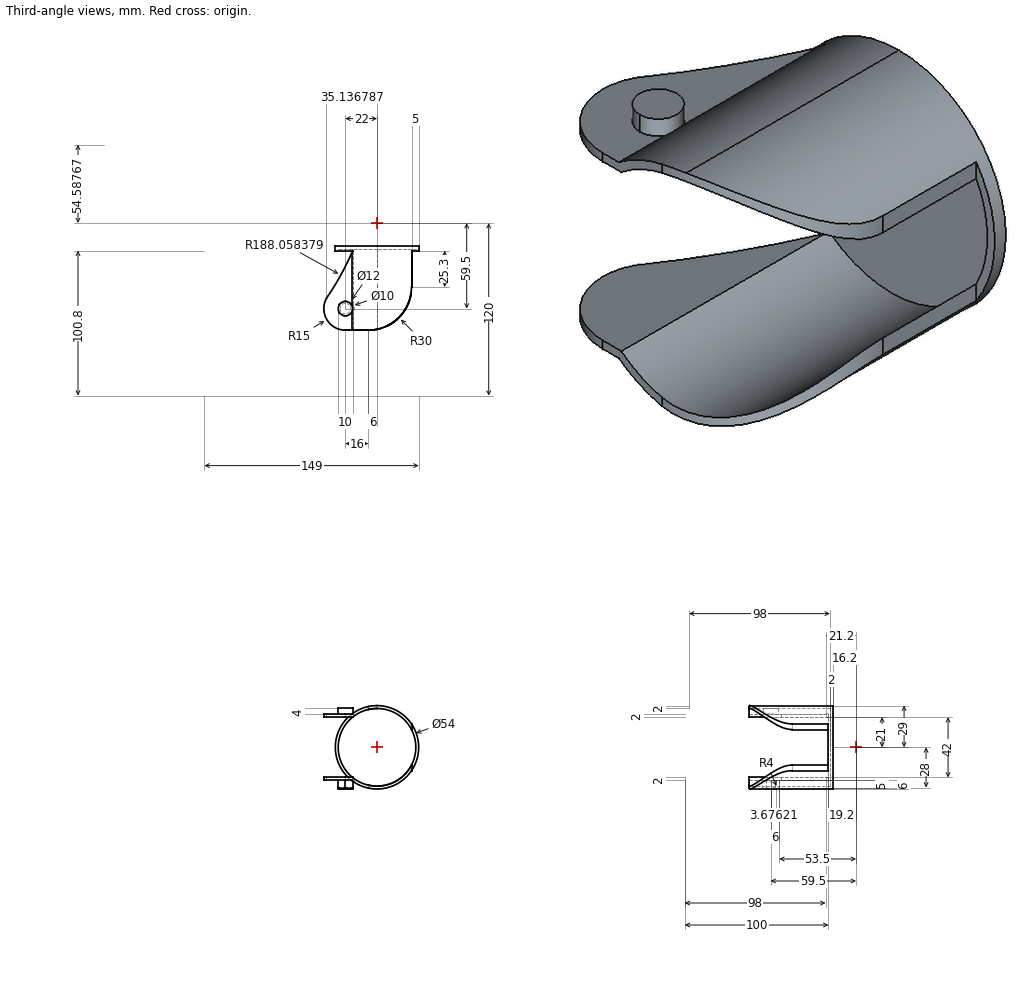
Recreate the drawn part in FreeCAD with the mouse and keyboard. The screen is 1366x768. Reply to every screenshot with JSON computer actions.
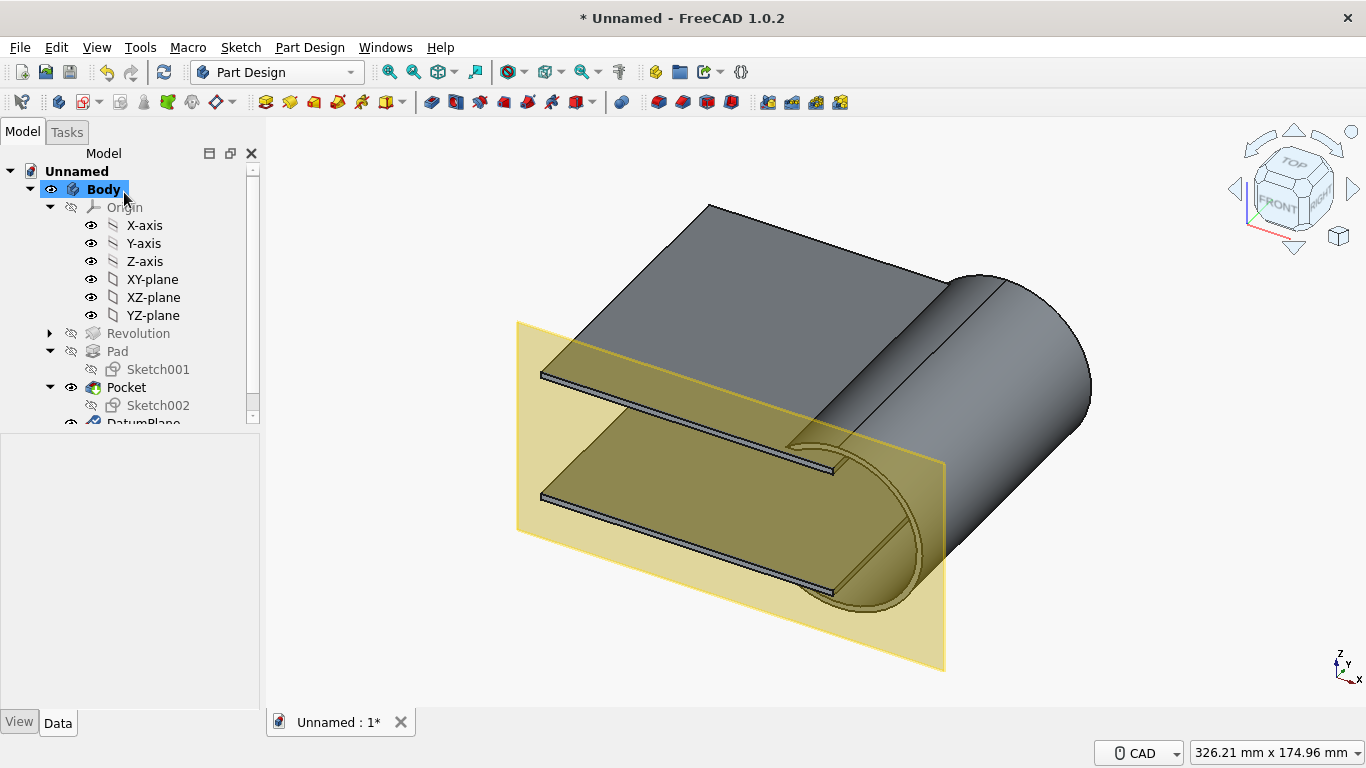
{"action": "left_click", "coordinate": [116, 423]}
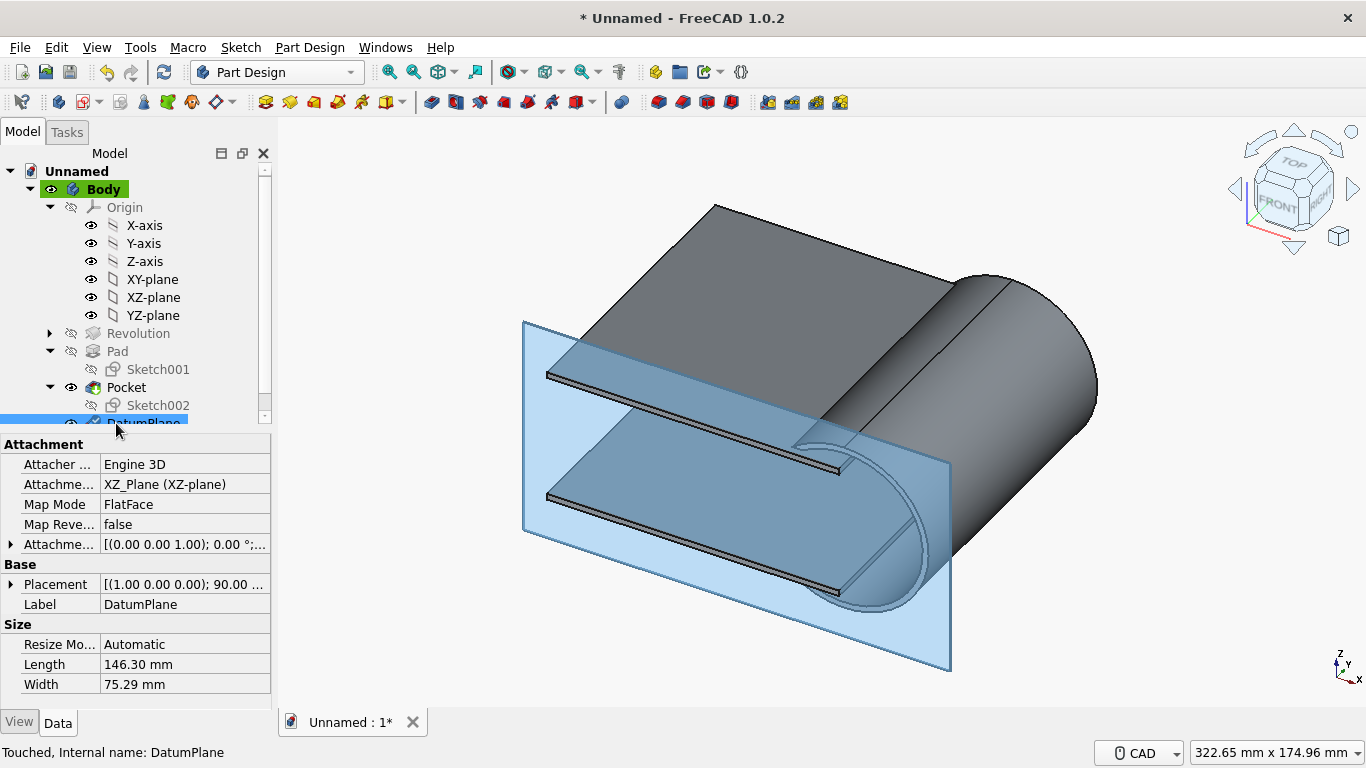
{"action": "left_click", "coordinate": [84, 102]}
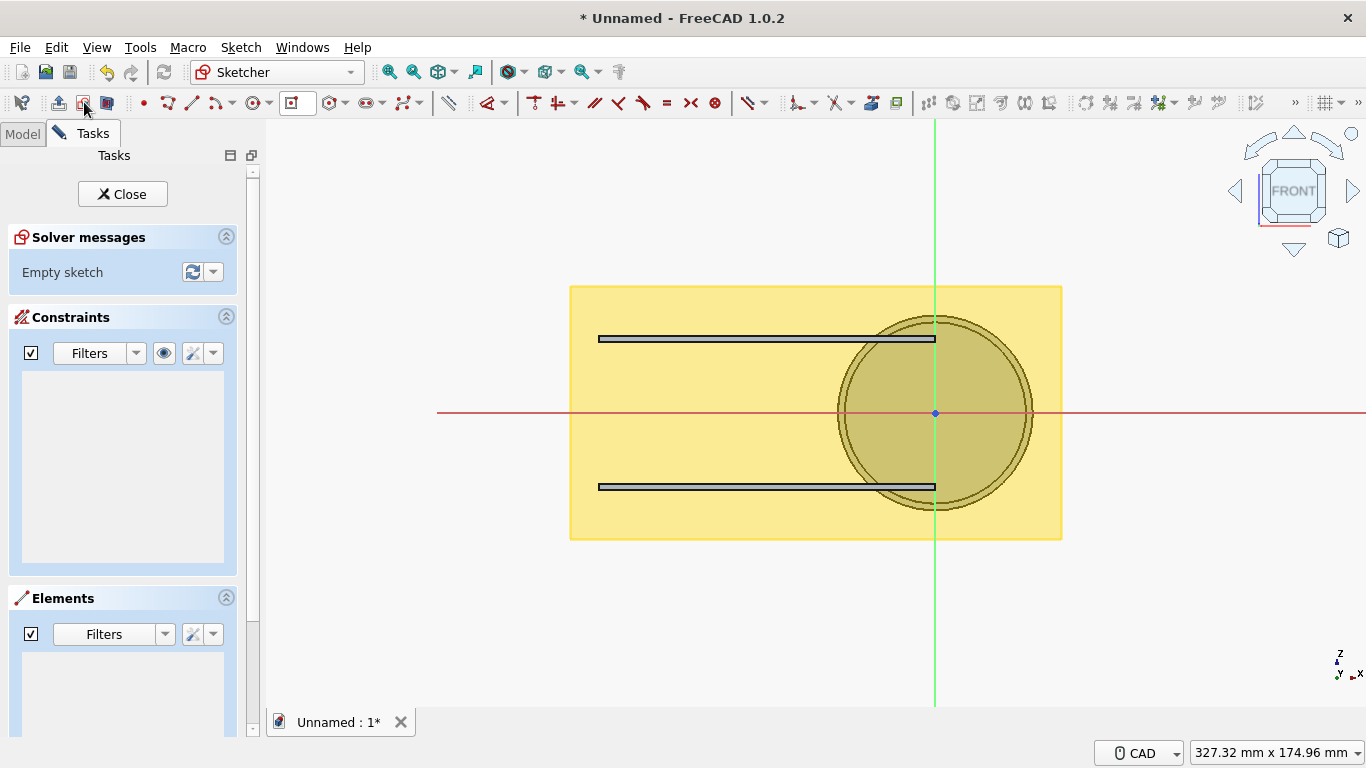
{"action": "left_click", "coordinate": [108, 104]}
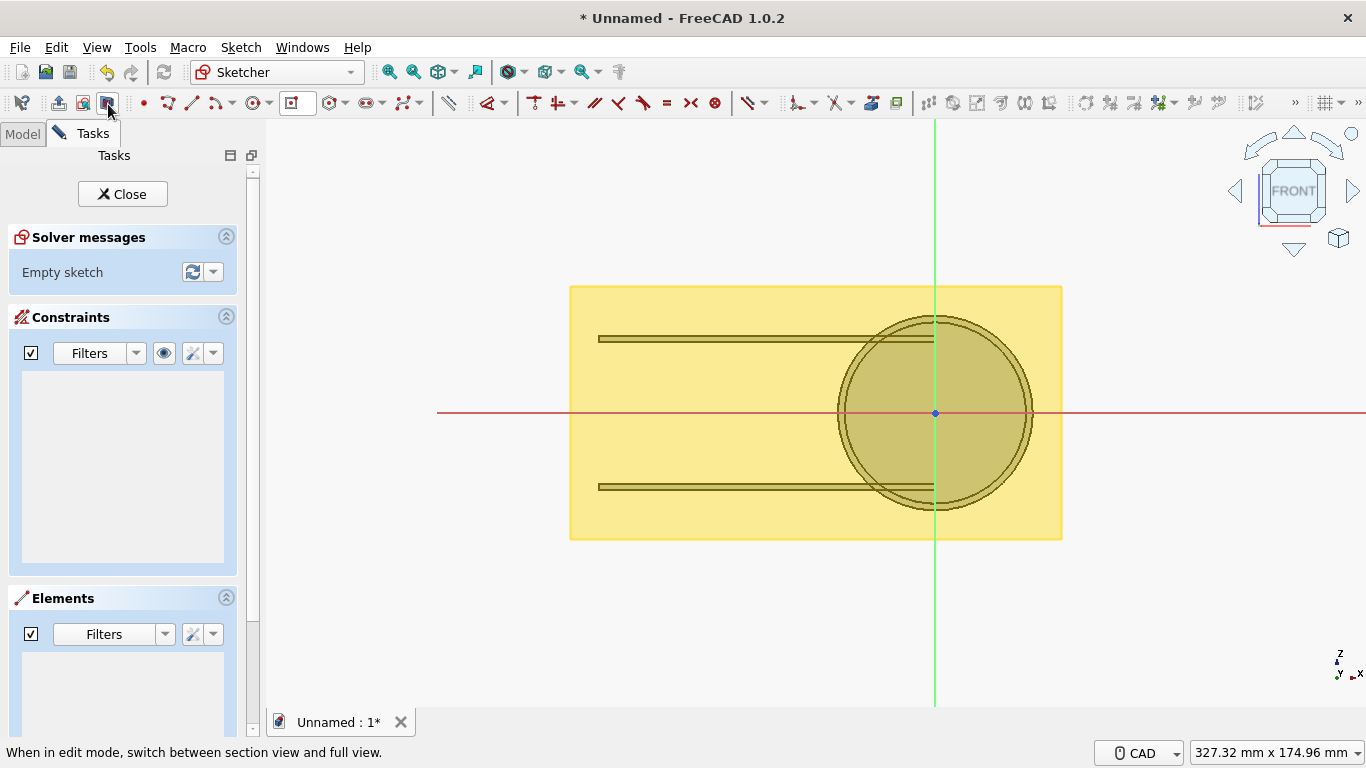
{"action": "scroll", "coordinate": [1089, 413], "scroll_direction": "up", "scroll_amount": 4}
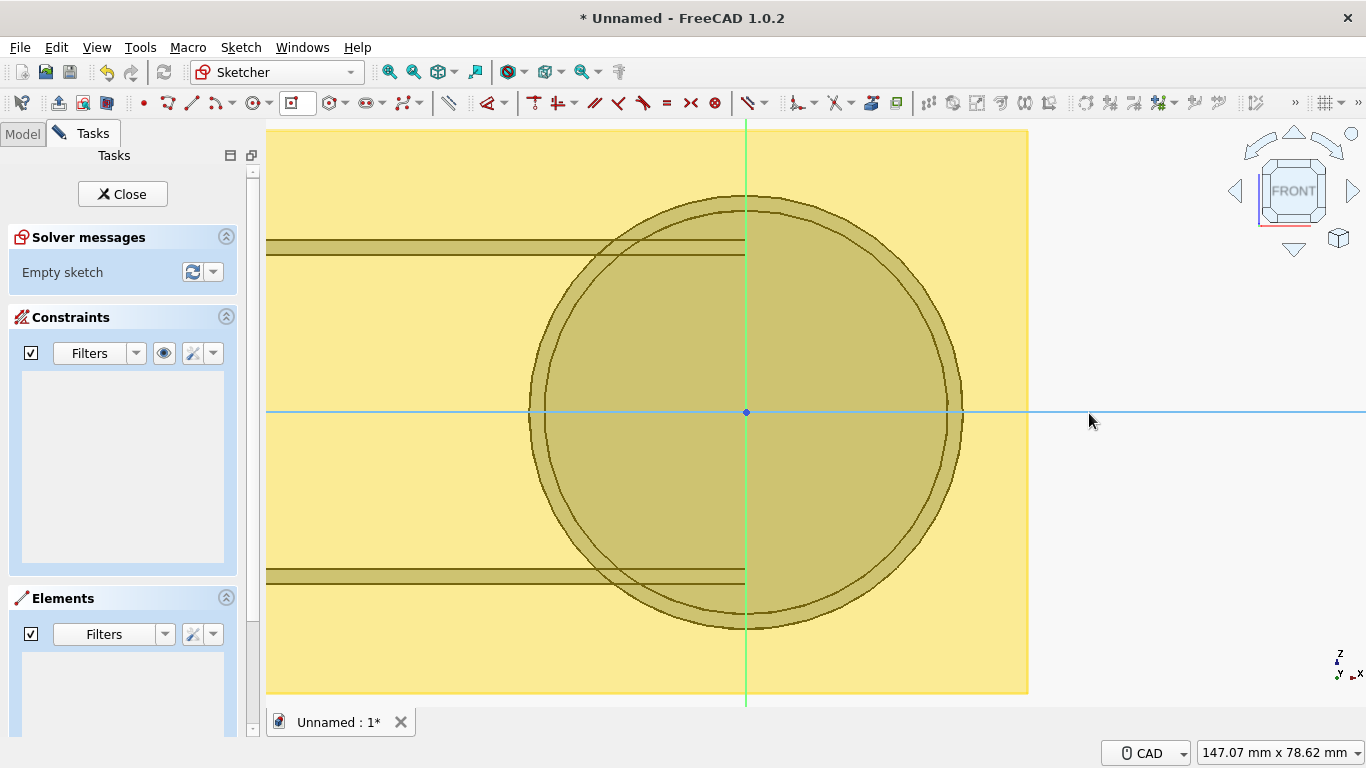
{"action": "left_click", "coordinate": [254, 104]}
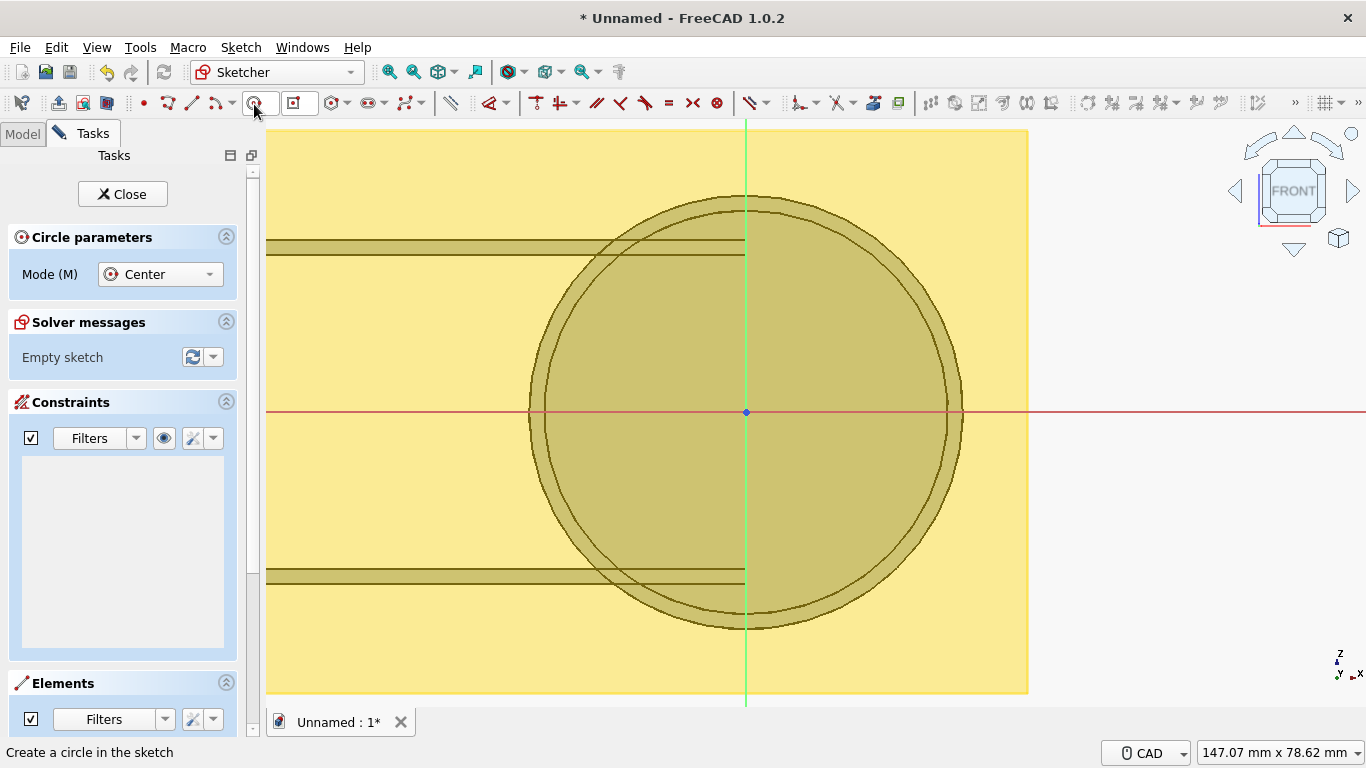
{"action": "left_click", "coordinate": [746, 412]}
{"action": "left_click", "coordinate": [889, 270]}
{"action": "key", "text": "Escape"}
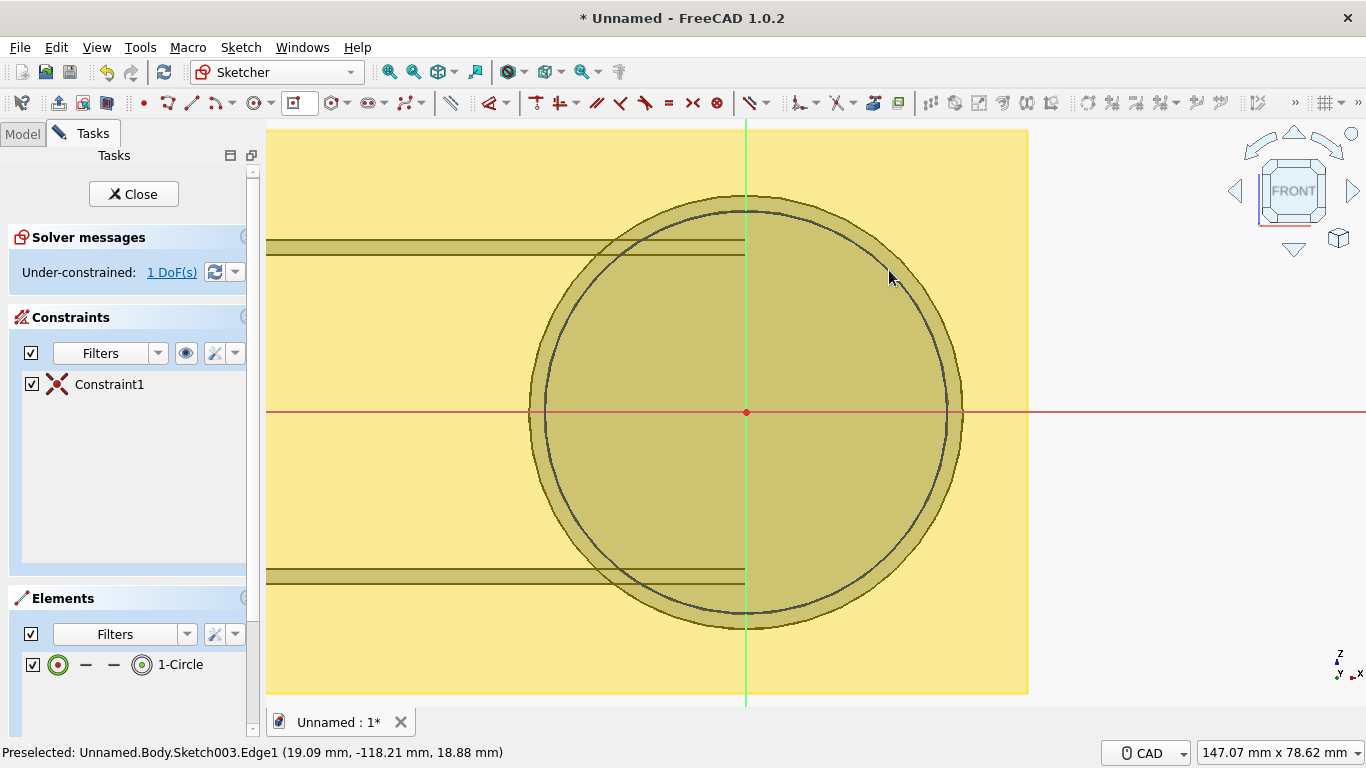
{"action": "left_click", "coordinate": [490, 104]}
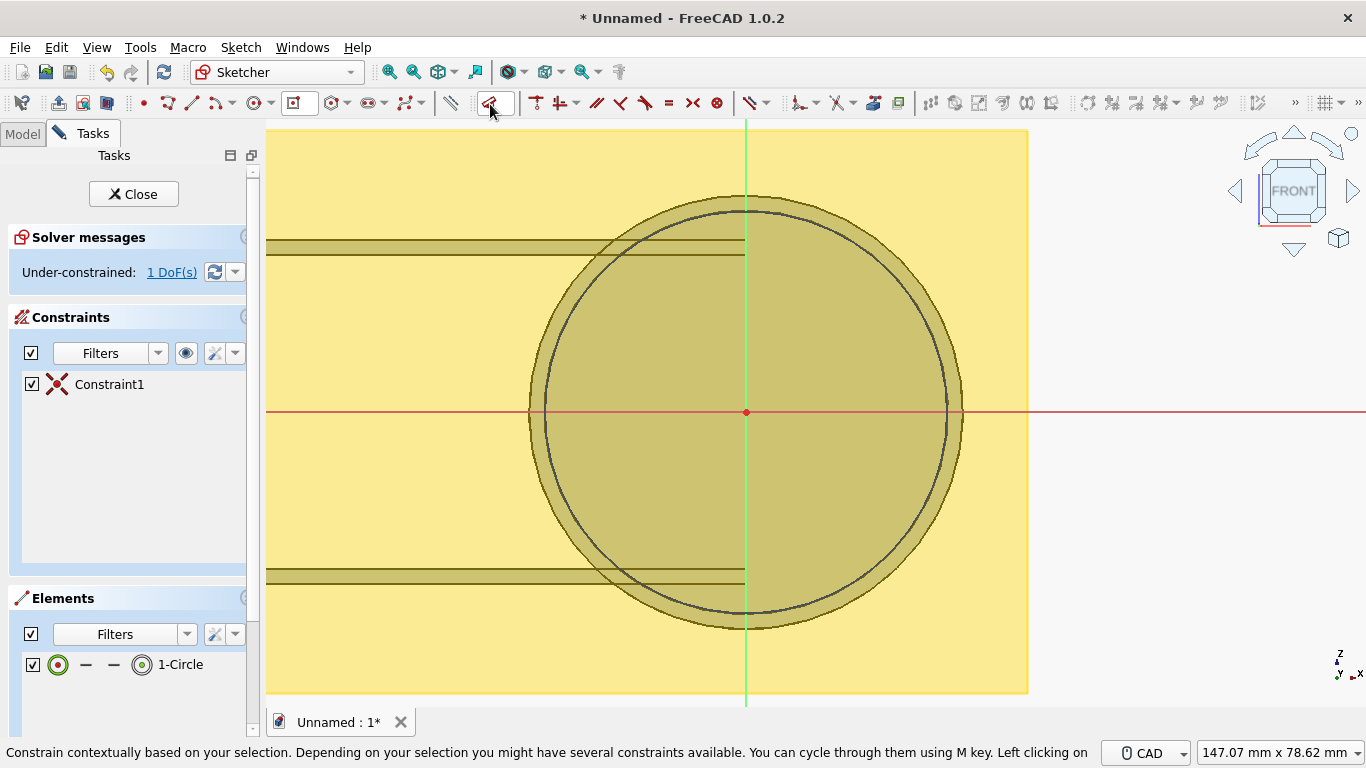
{"action": "left_click", "coordinate": [888, 270]}
{"action": "left_click", "coordinate": [911, 247]}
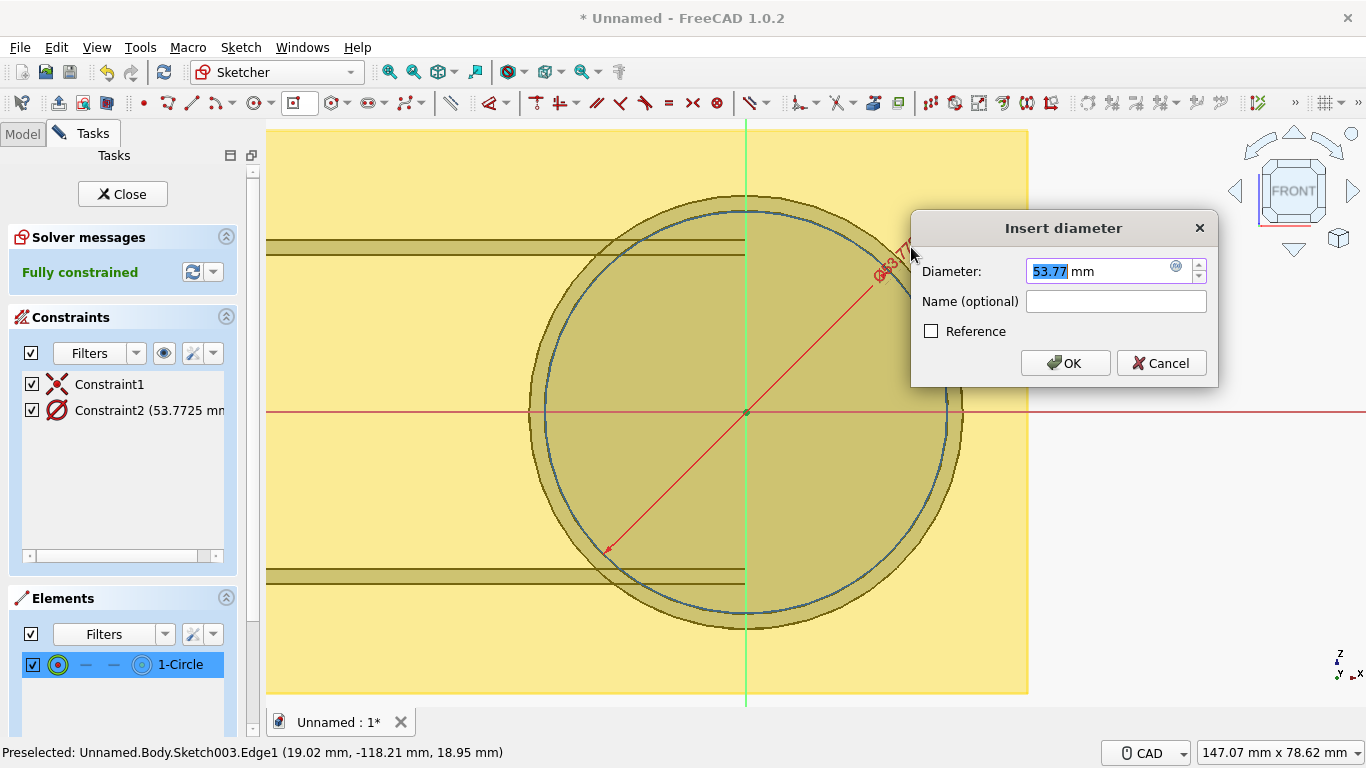
{"action": "type", "text": "54"}
{"action": "key", "text": "Return"}
{"action": "key", "text": "Escape"}